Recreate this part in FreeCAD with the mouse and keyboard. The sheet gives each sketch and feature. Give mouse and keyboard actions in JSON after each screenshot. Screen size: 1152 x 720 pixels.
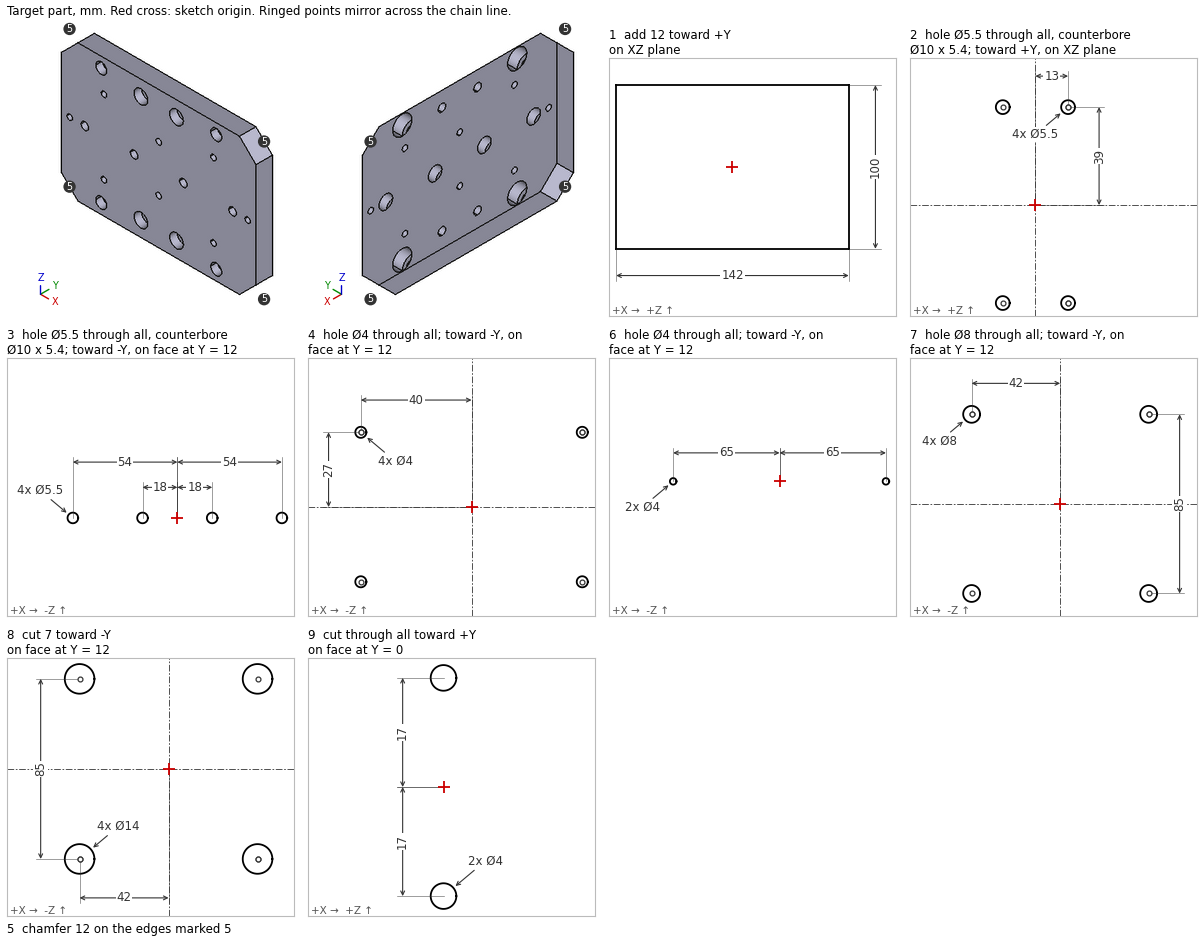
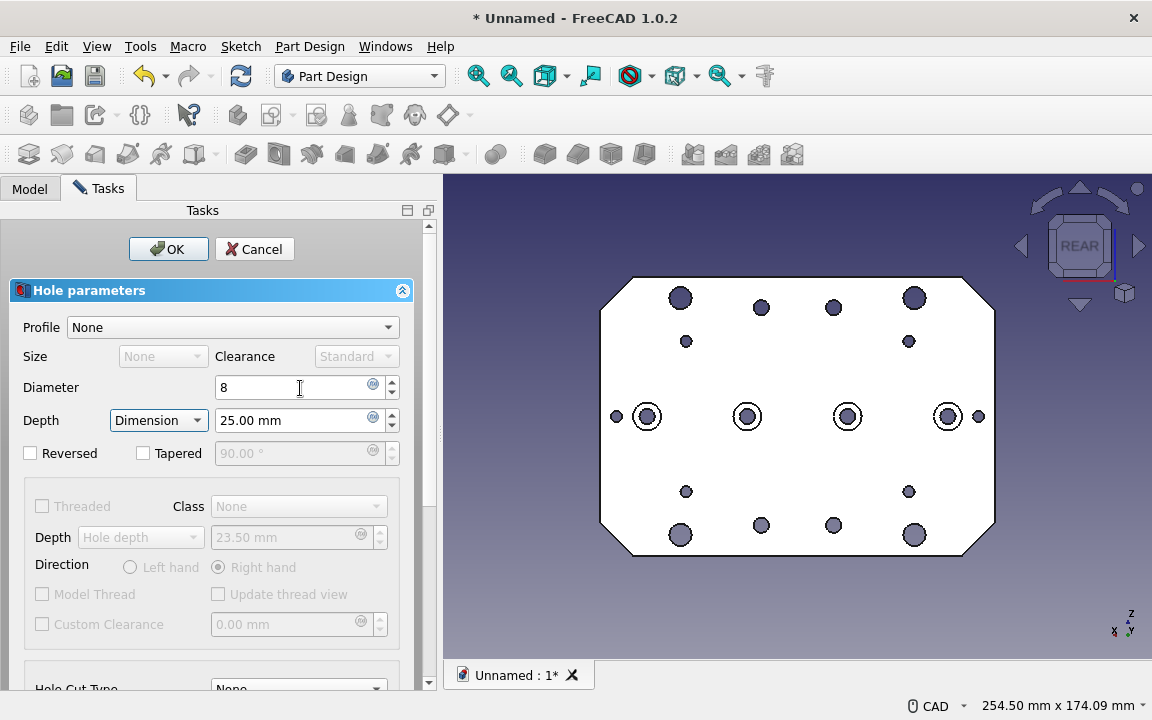
{"action": "left_click", "coordinate": [160, 420]}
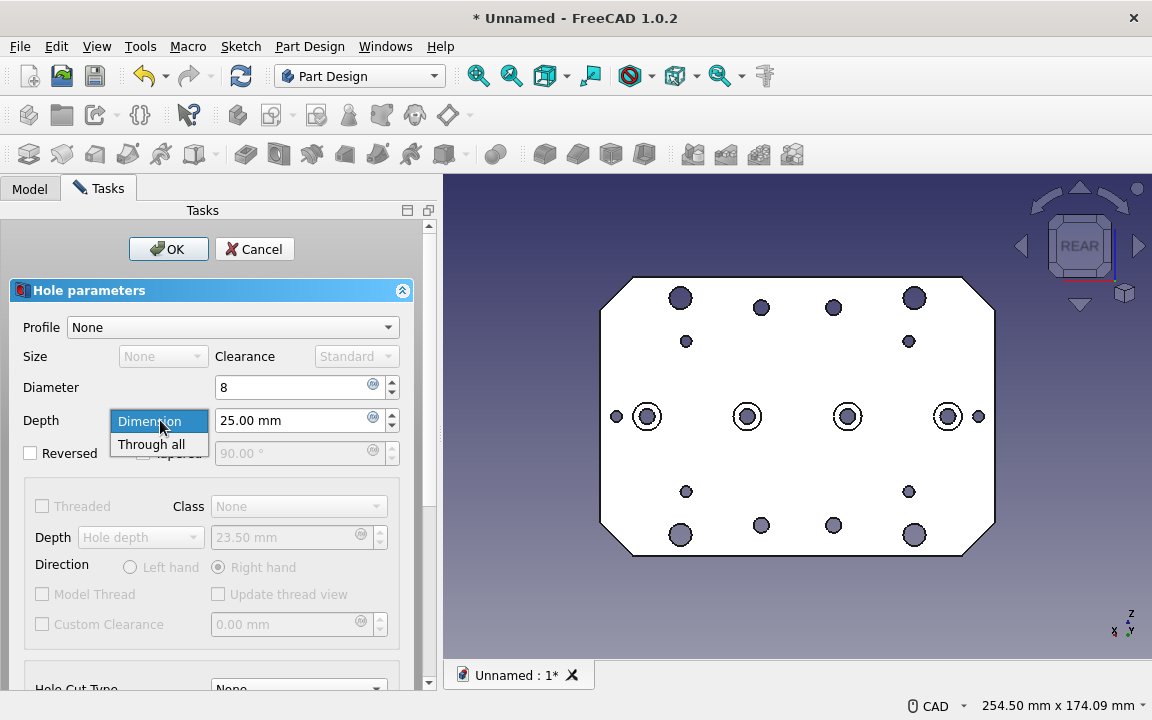
{"action": "left_click", "coordinate": [158, 444]}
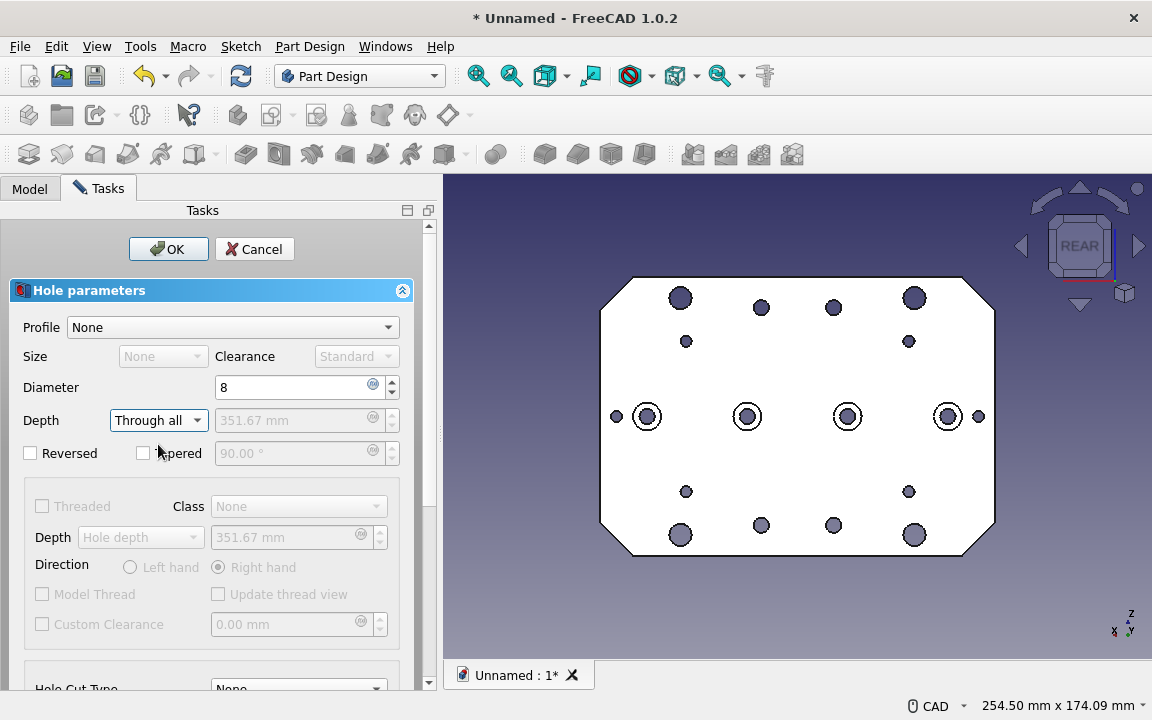
{"action": "left_click", "coordinate": [169, 249]}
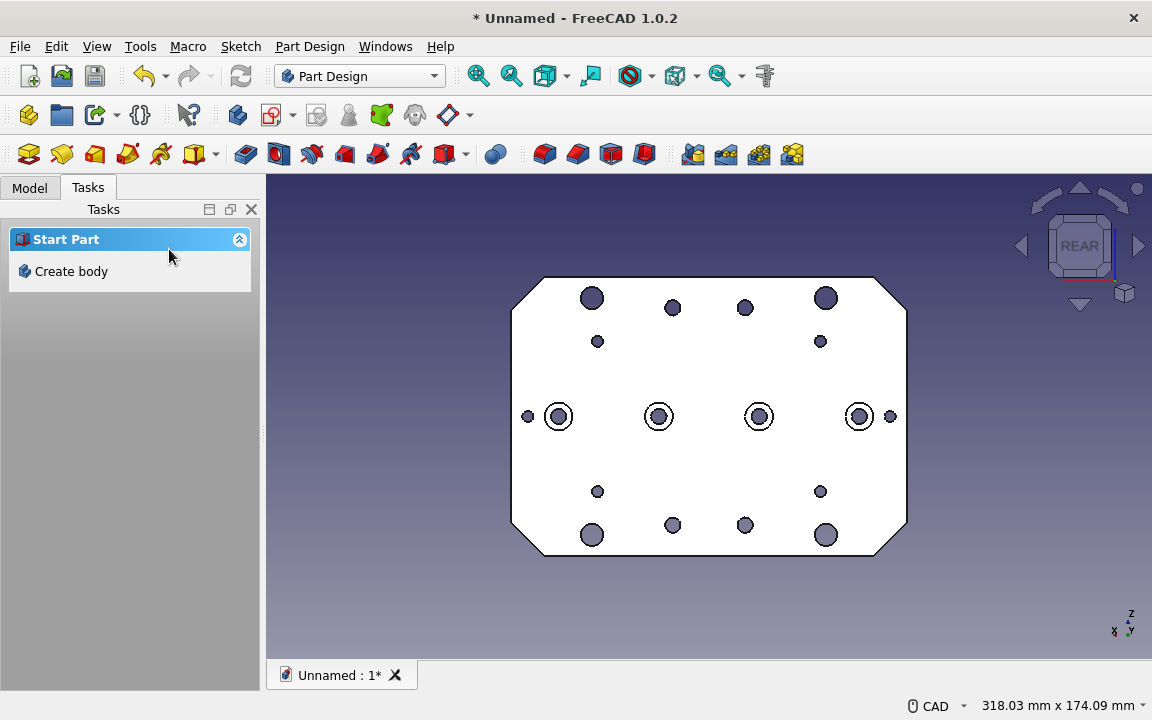
{"action": "left_click", "coordinate": [709, 455]}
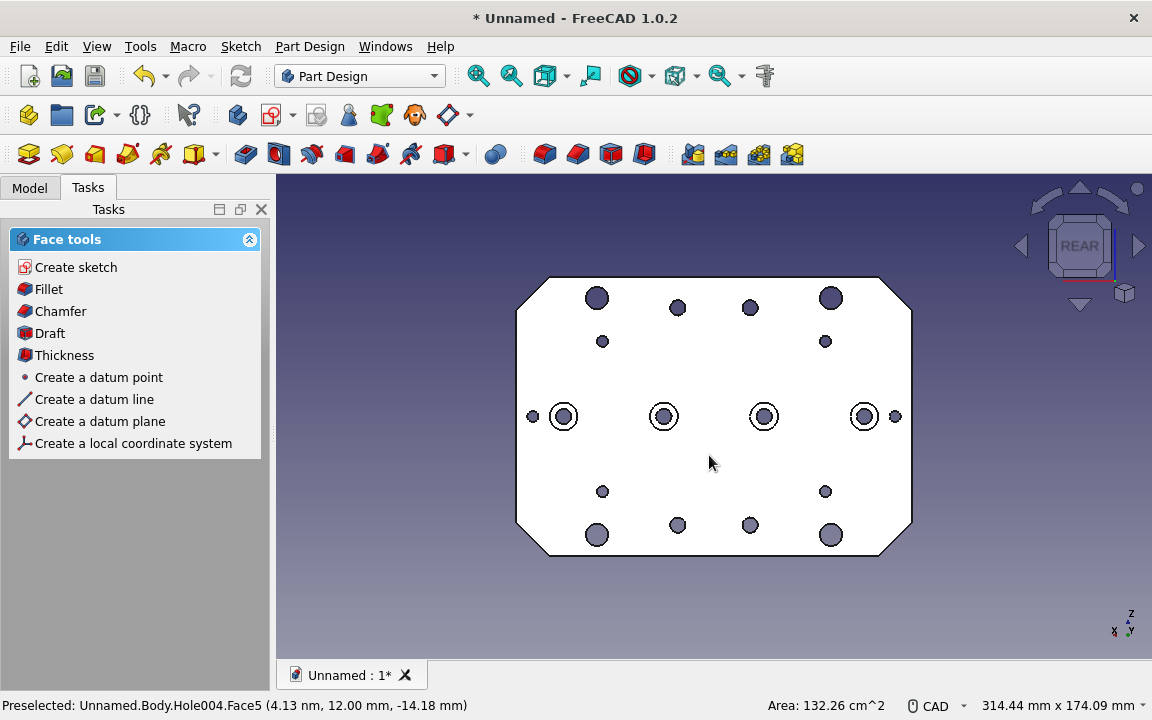
{"action": "left_click", "coordinate": [270, 116]}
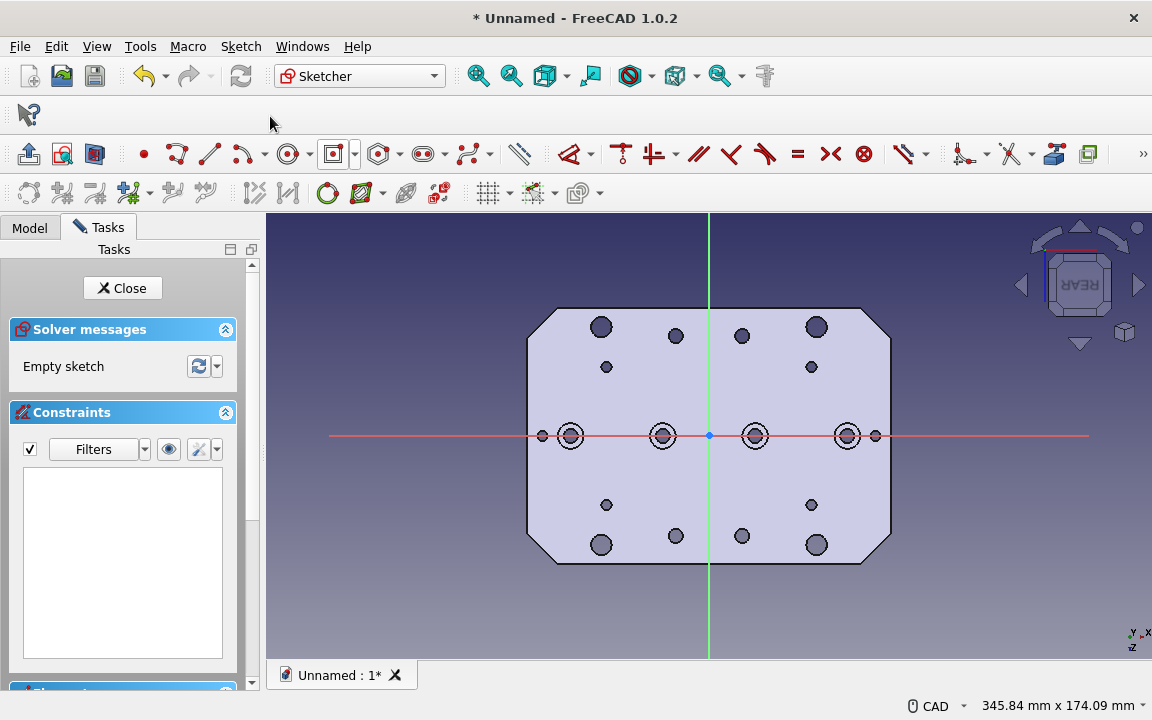
{"action": "left_click", "coordinate": [288, 154]}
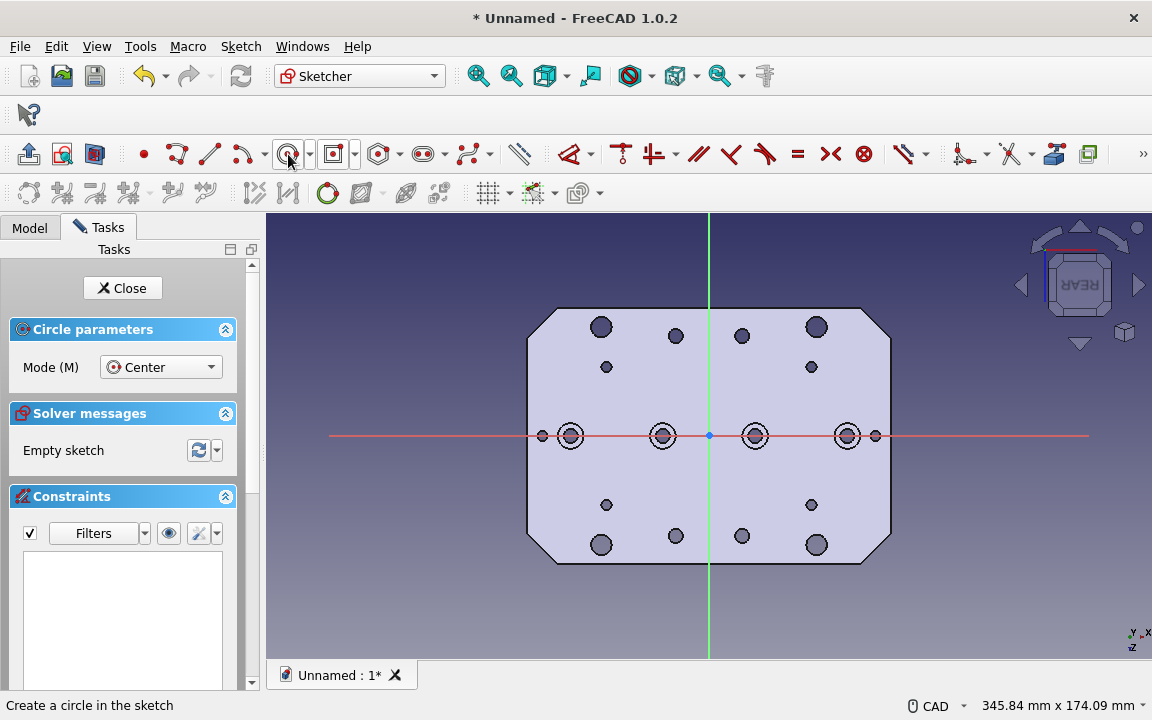
{"action": "scroll", "coordinate": [601, 545], "scroll_direction": "up", "scroll_amount": 2}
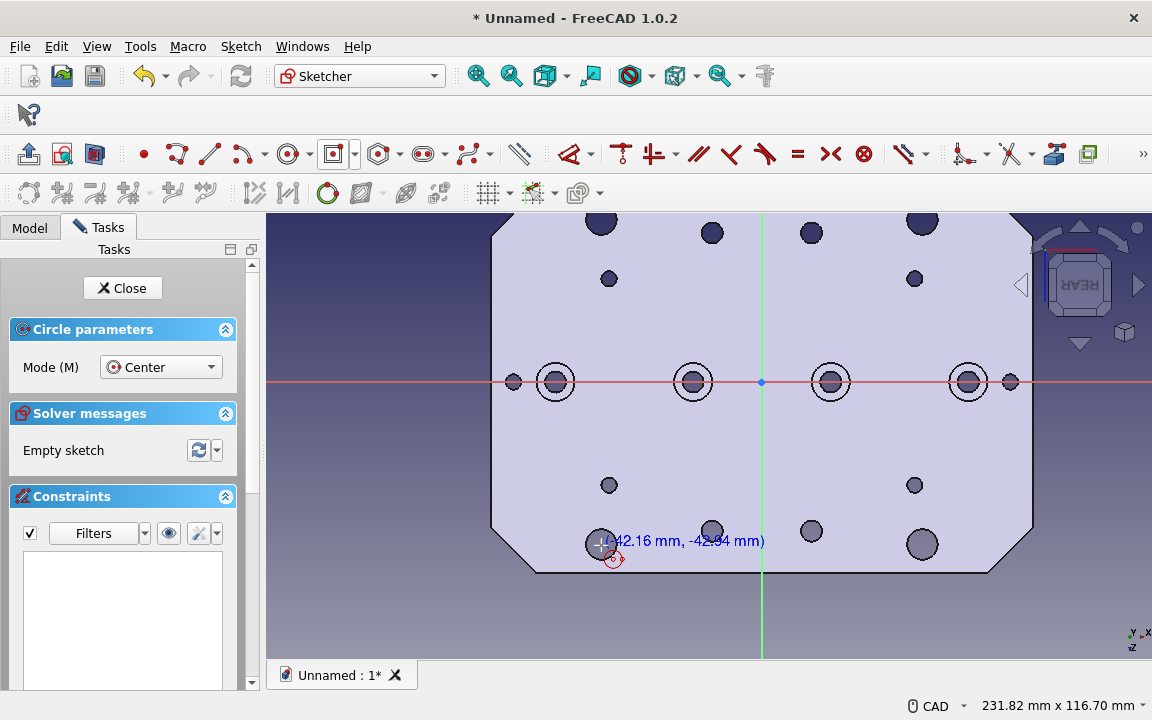
{"action": "left_click", "coordinate": [601, 544]}
{"action": "left_click", "coordinate": [620, 526]}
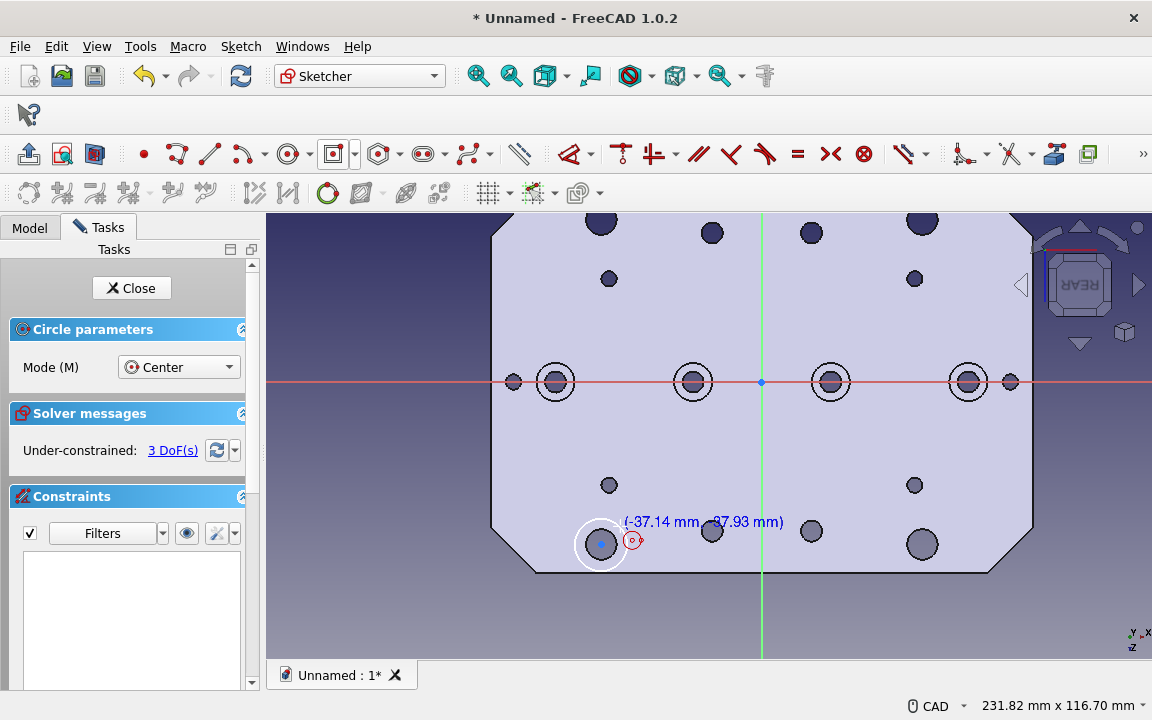
{"action": "left_click", "coordinate": [922, 544]}
{"action": "left_click", "coordinate": [941, 526]}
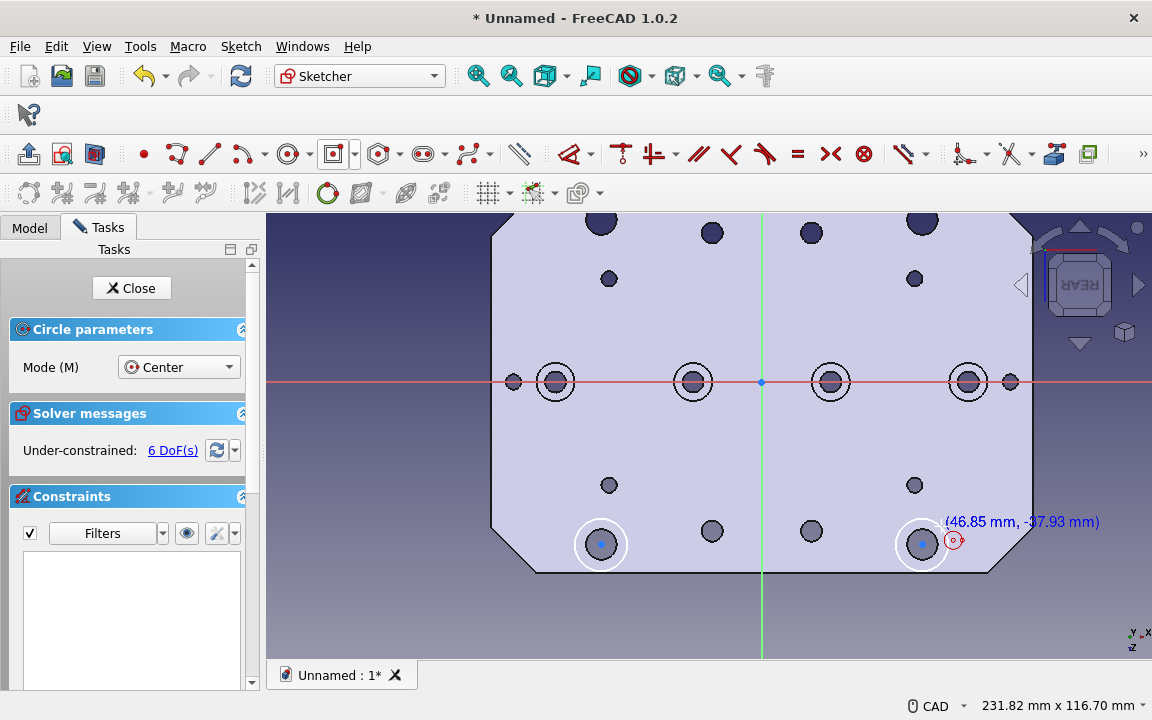
{"action": "scroll", "coordinate": [394, 546], "scroll_direction": "down", "scroll_amount": 2}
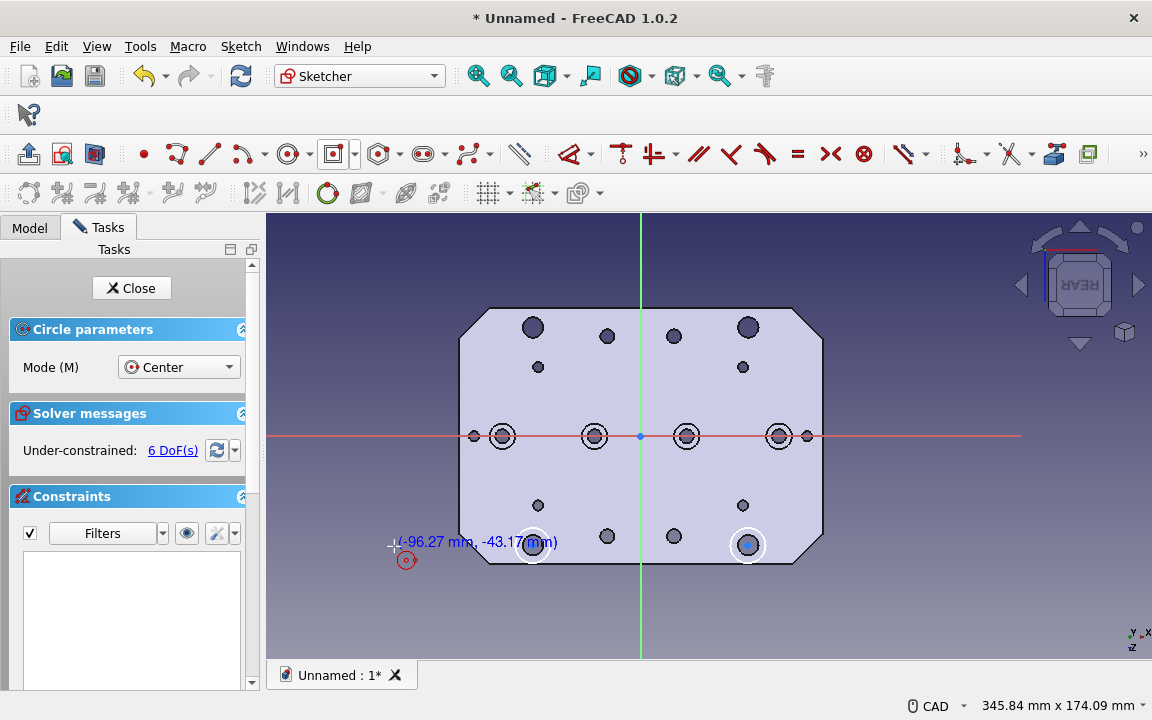
{"action": "scroll", "coordinate": [533, 327], "scroll_direction": "up", "scroll_amount": 2}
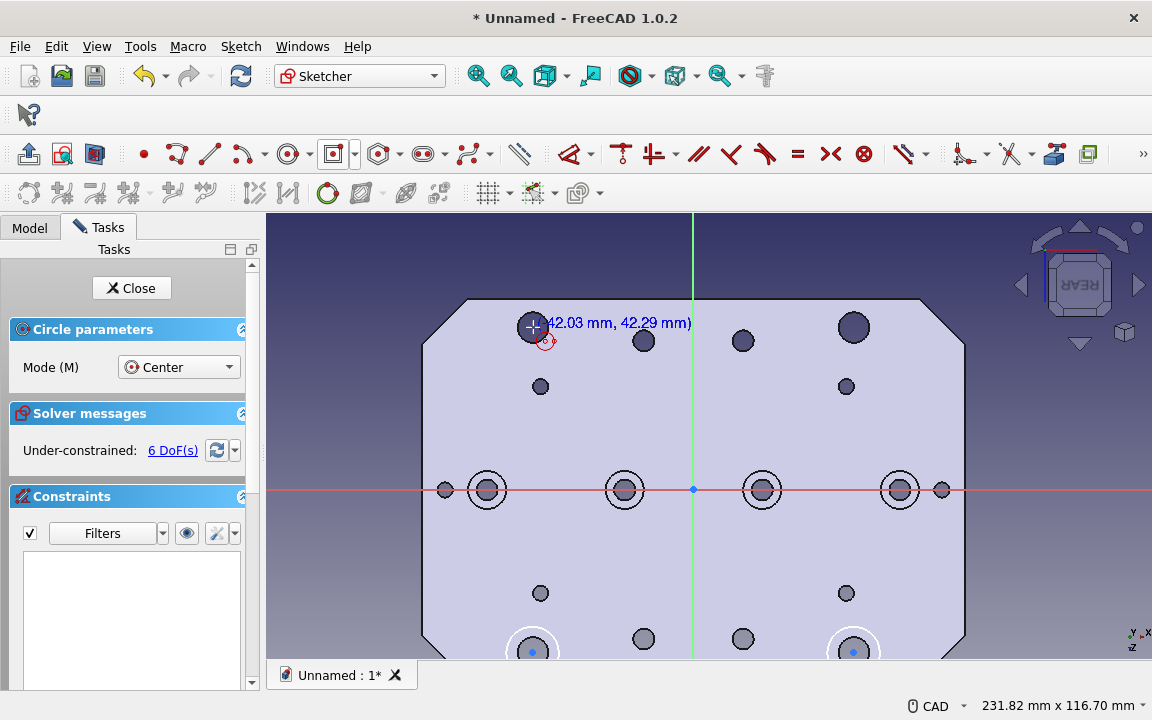
{"action": "left_click", "coordinate": [533, 328]}
{"action": "left_click", "coordinate": [552, 309]}